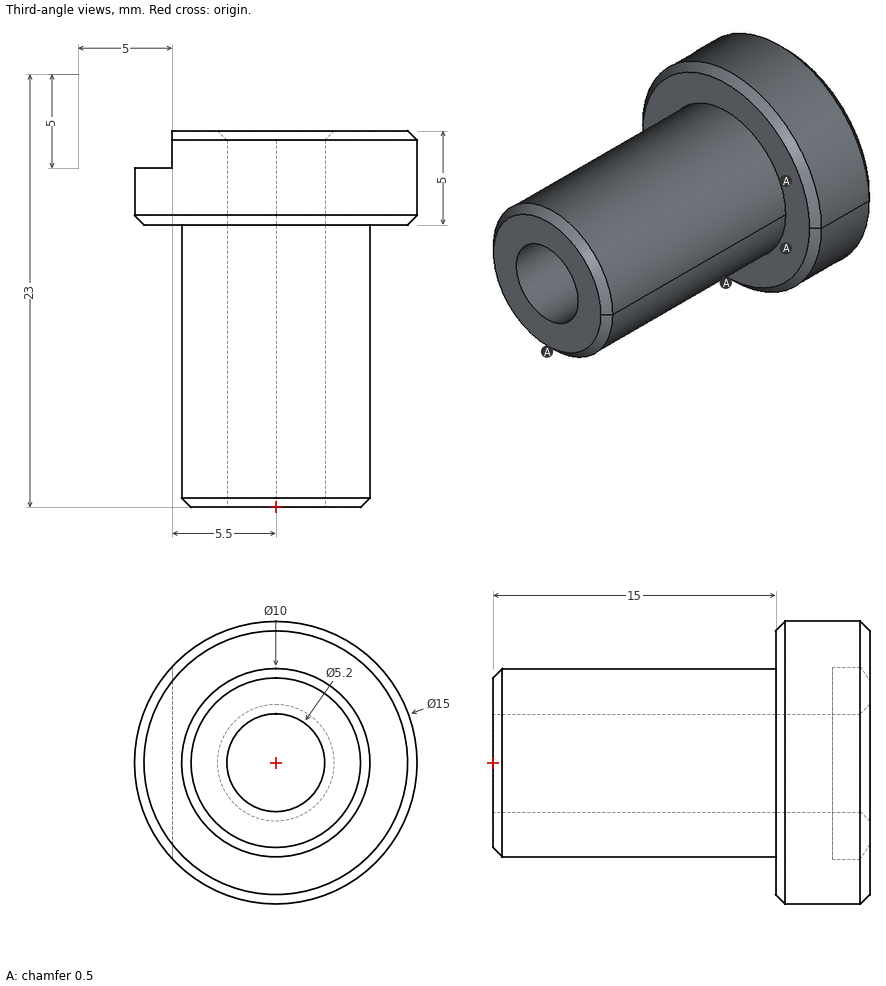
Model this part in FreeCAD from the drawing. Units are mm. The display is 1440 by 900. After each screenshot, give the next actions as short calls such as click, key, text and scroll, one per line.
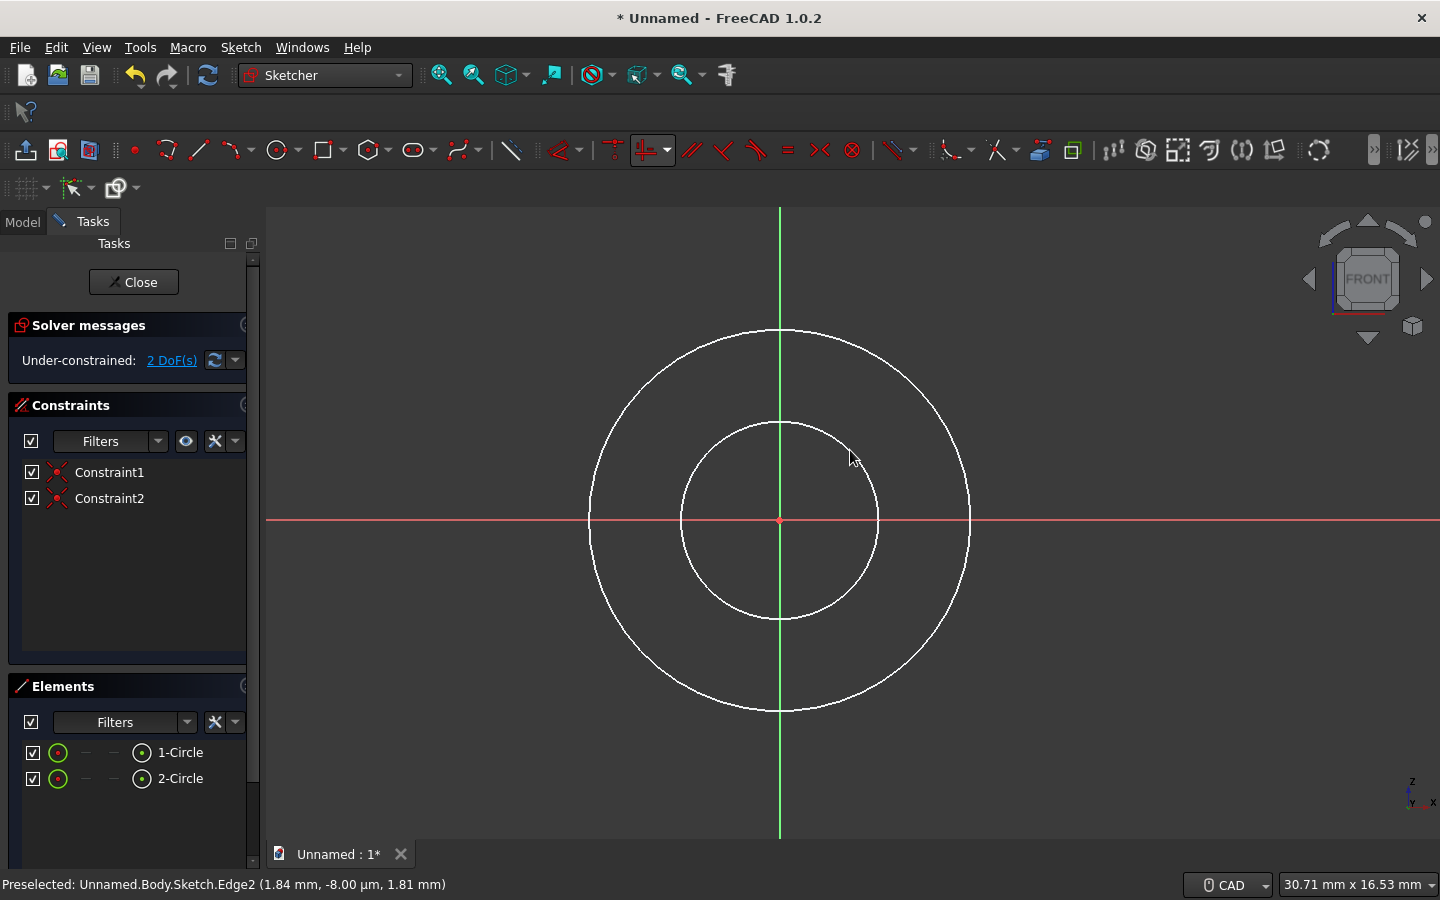
click(914, 385)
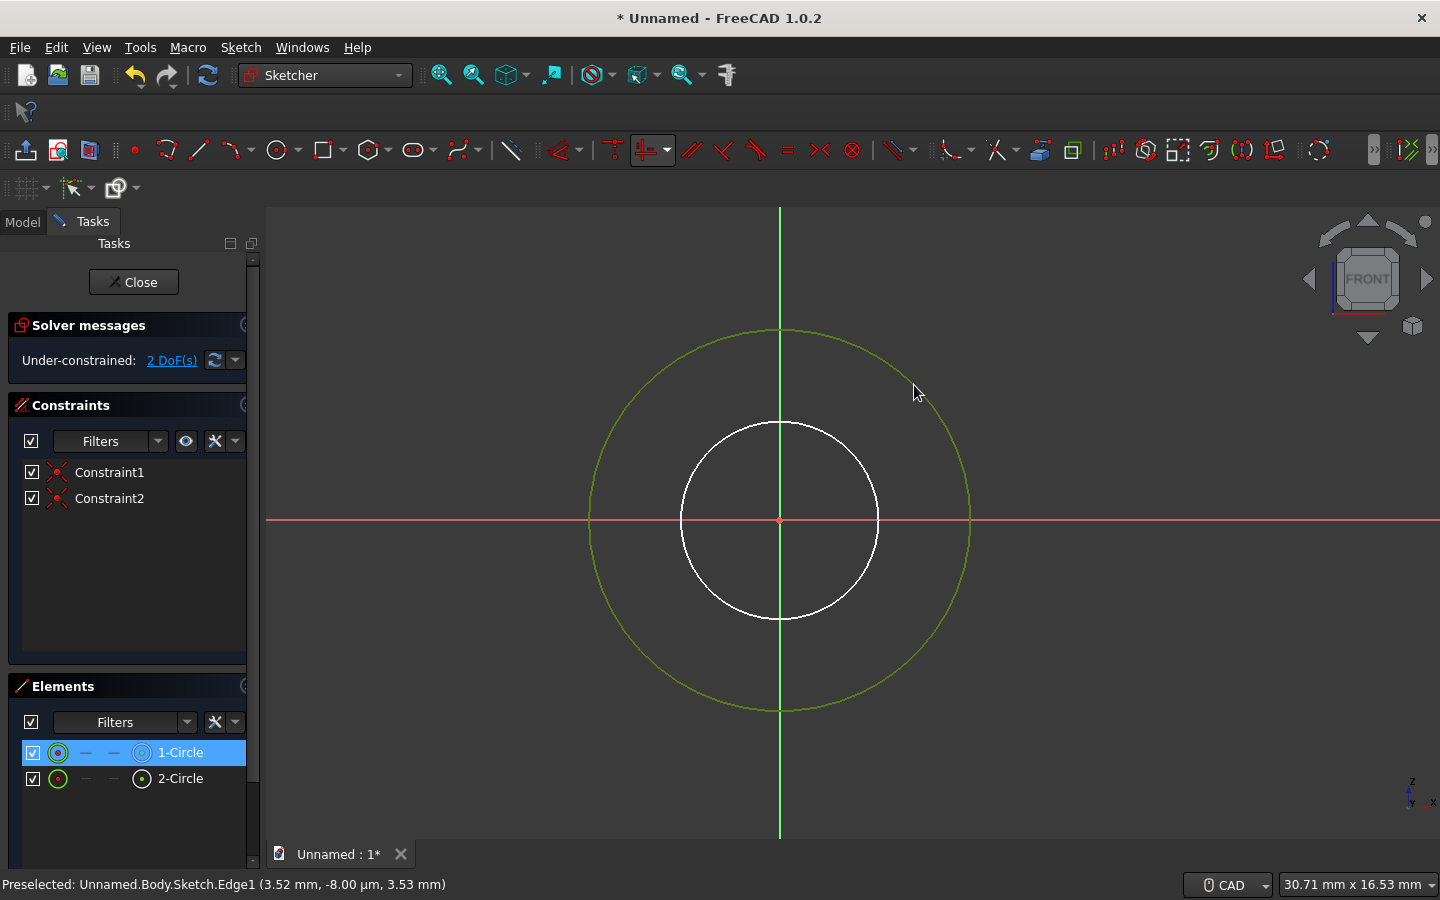
click(582, 150)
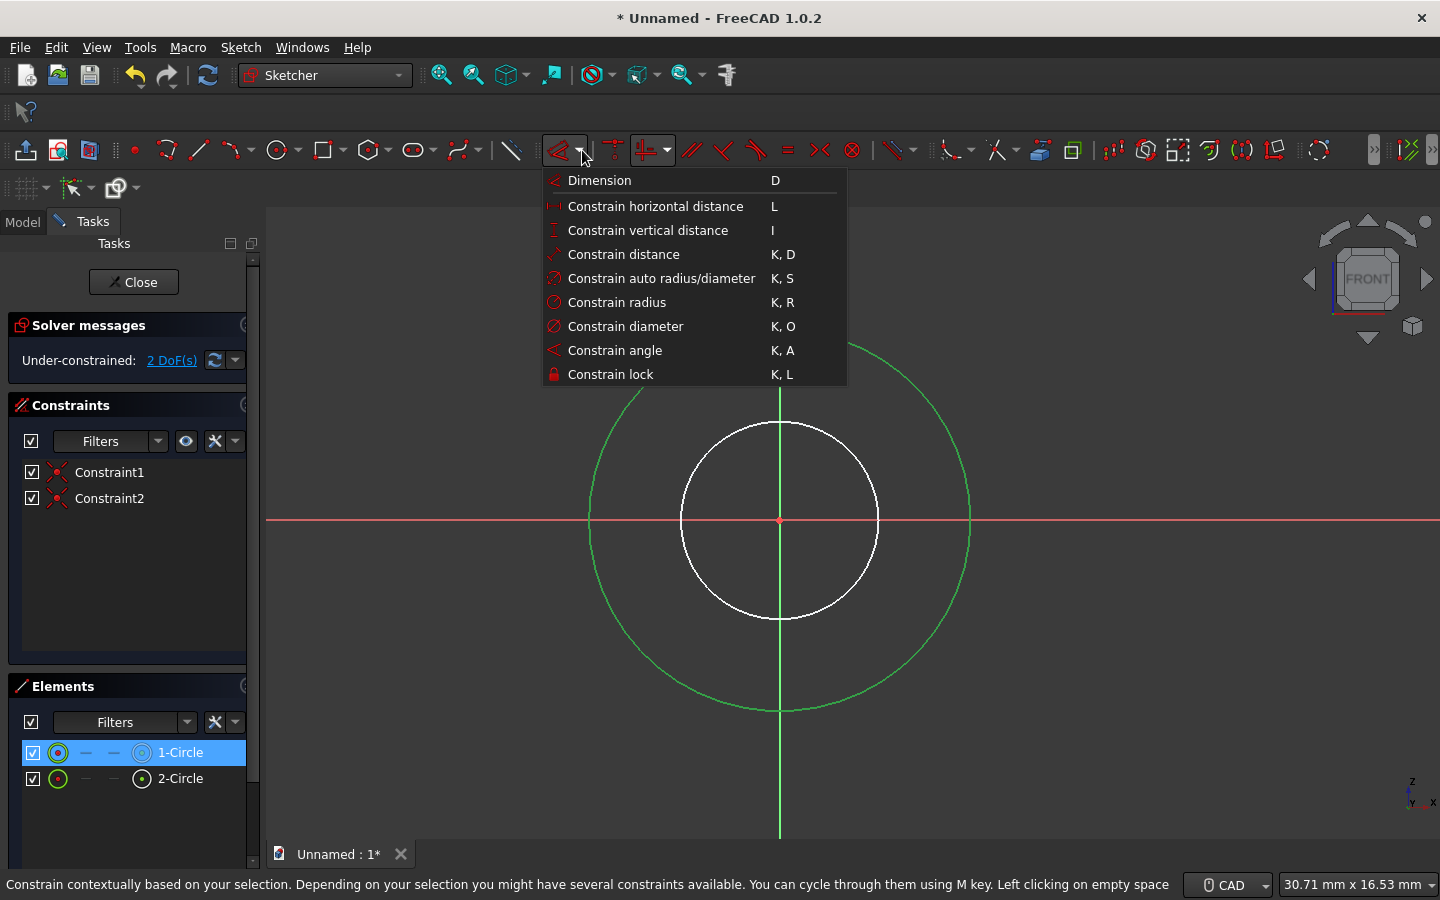
click(695, 326)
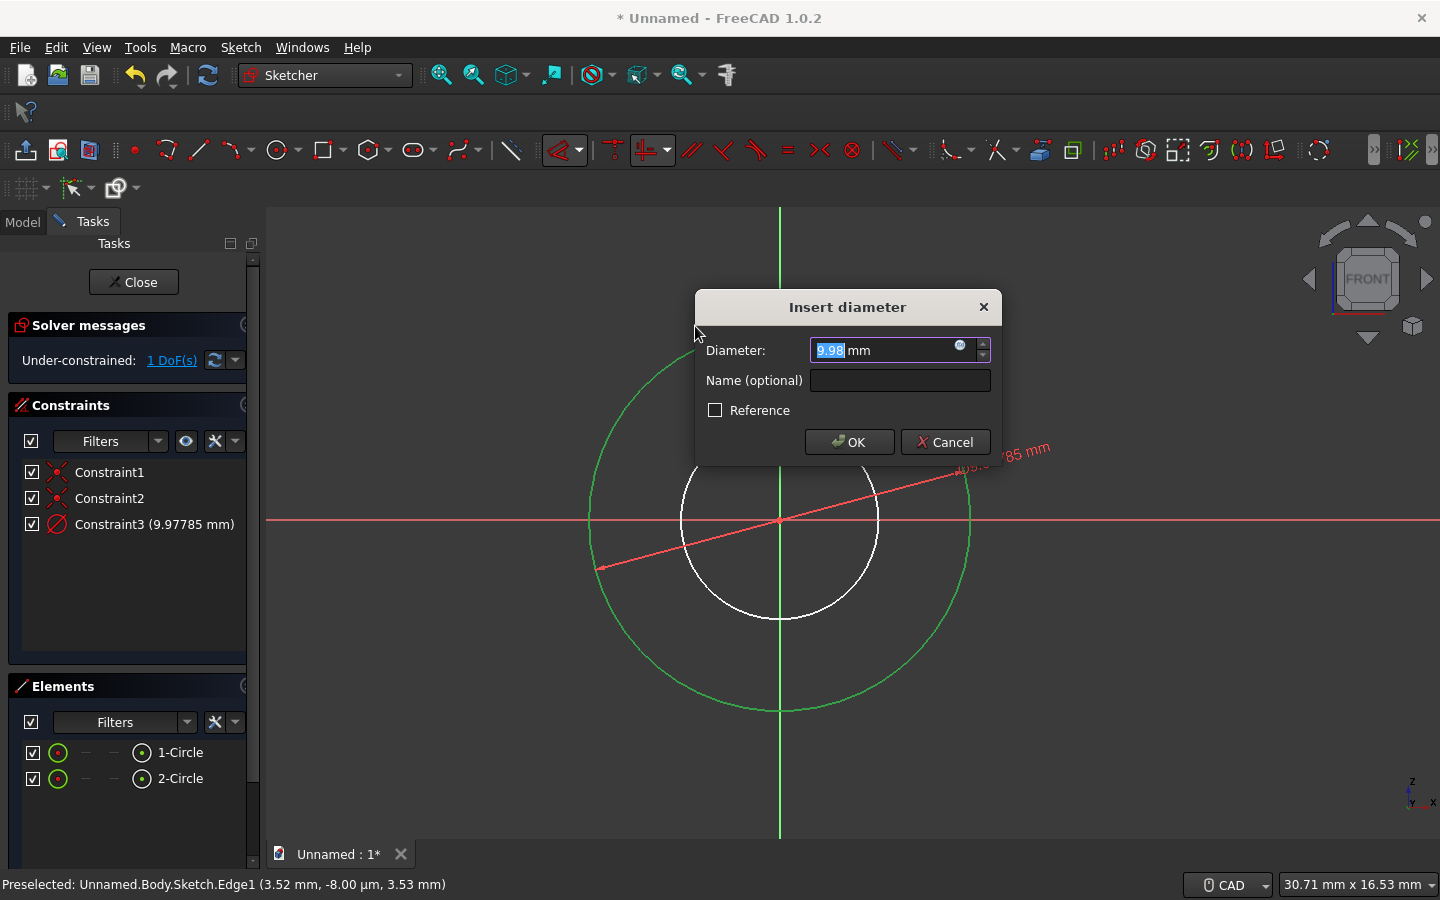
text(10)
key(Return)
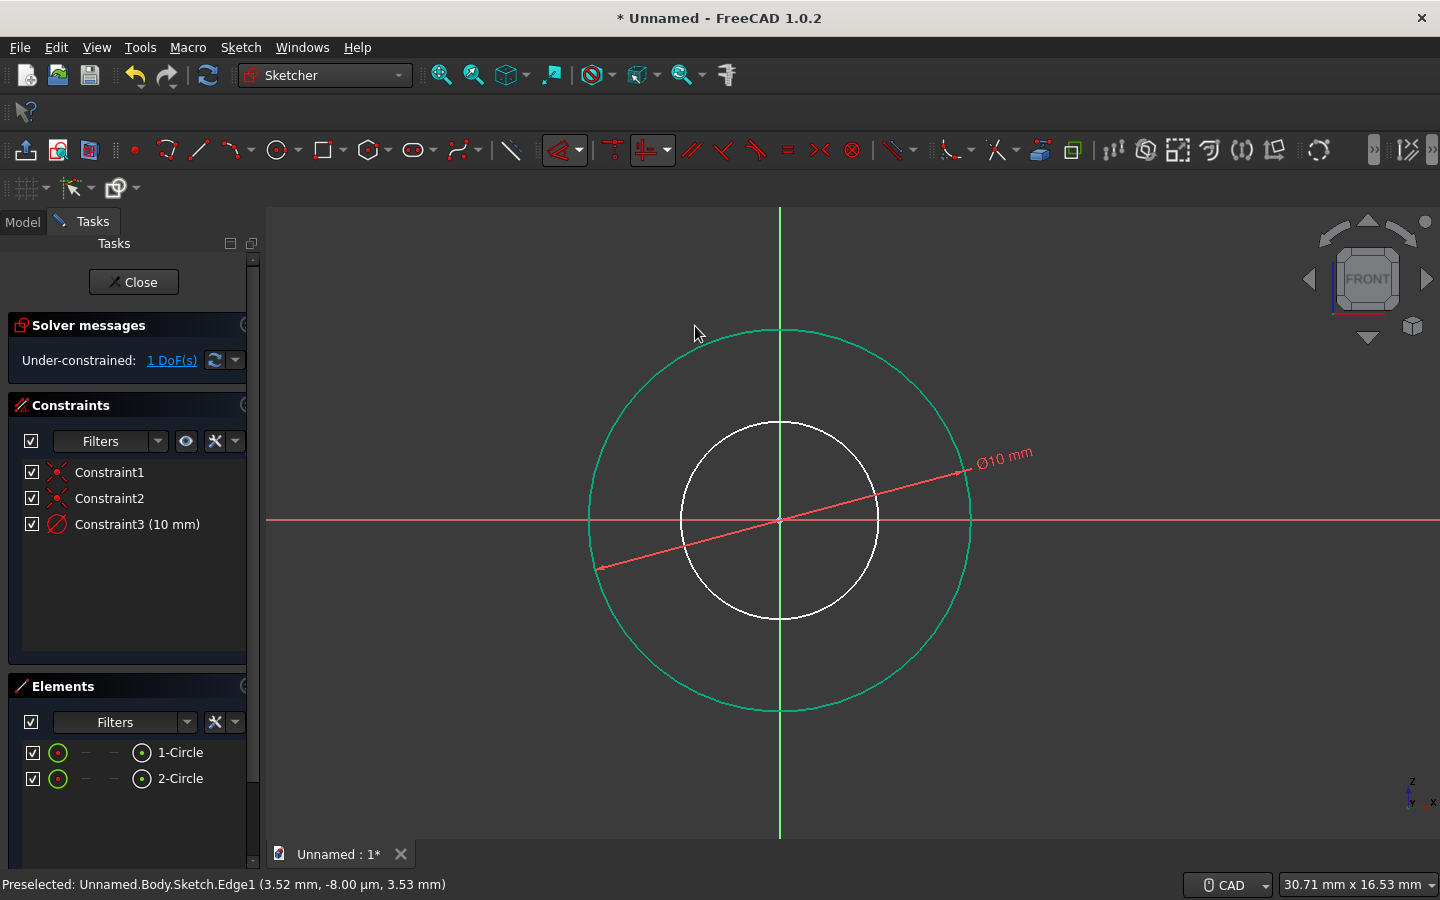
click(849, 450)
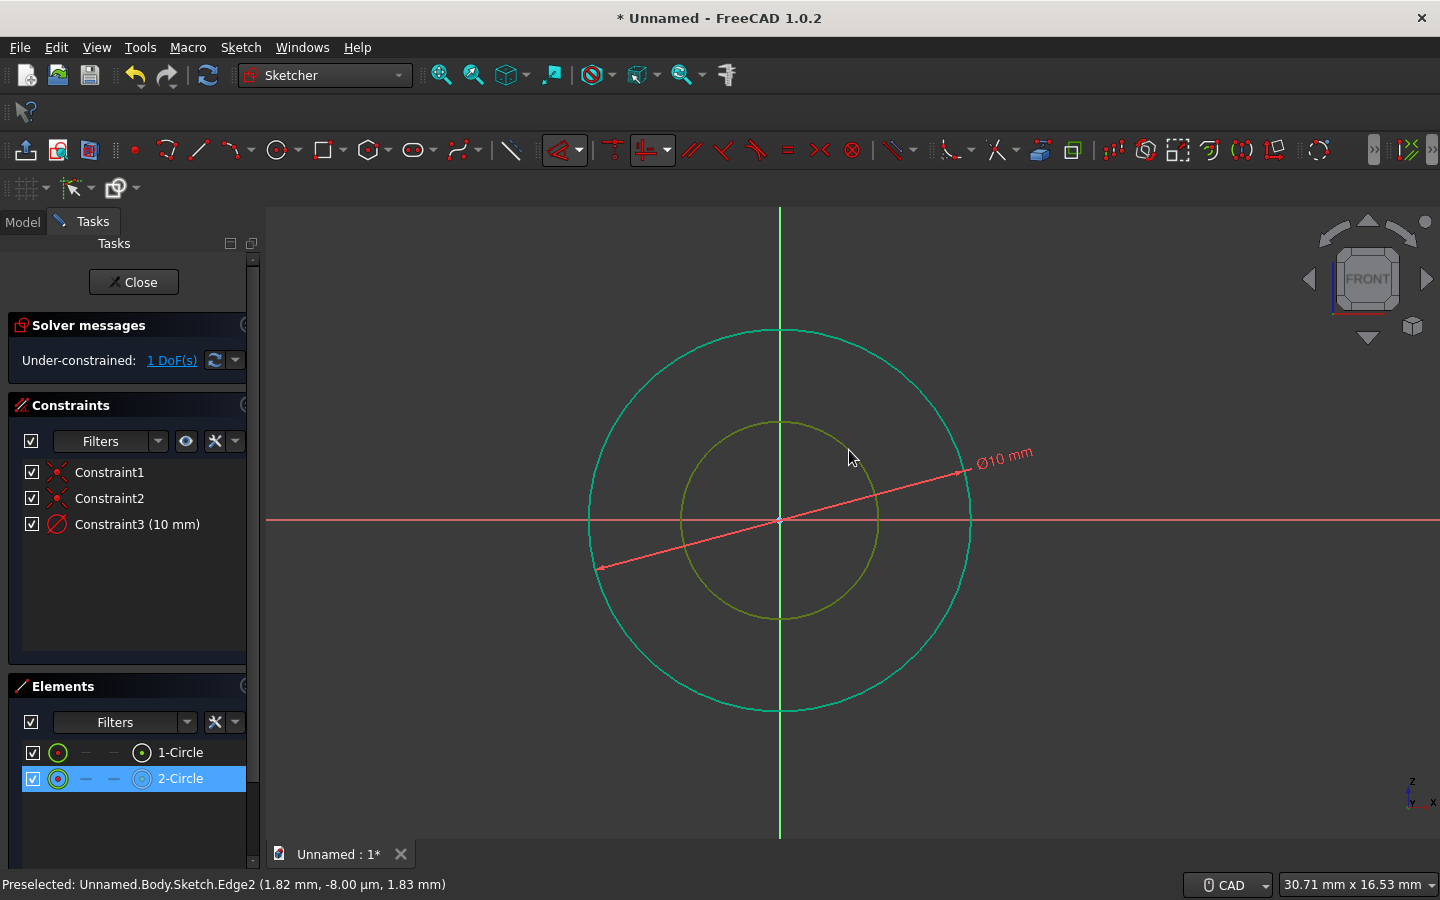
click(582, 150)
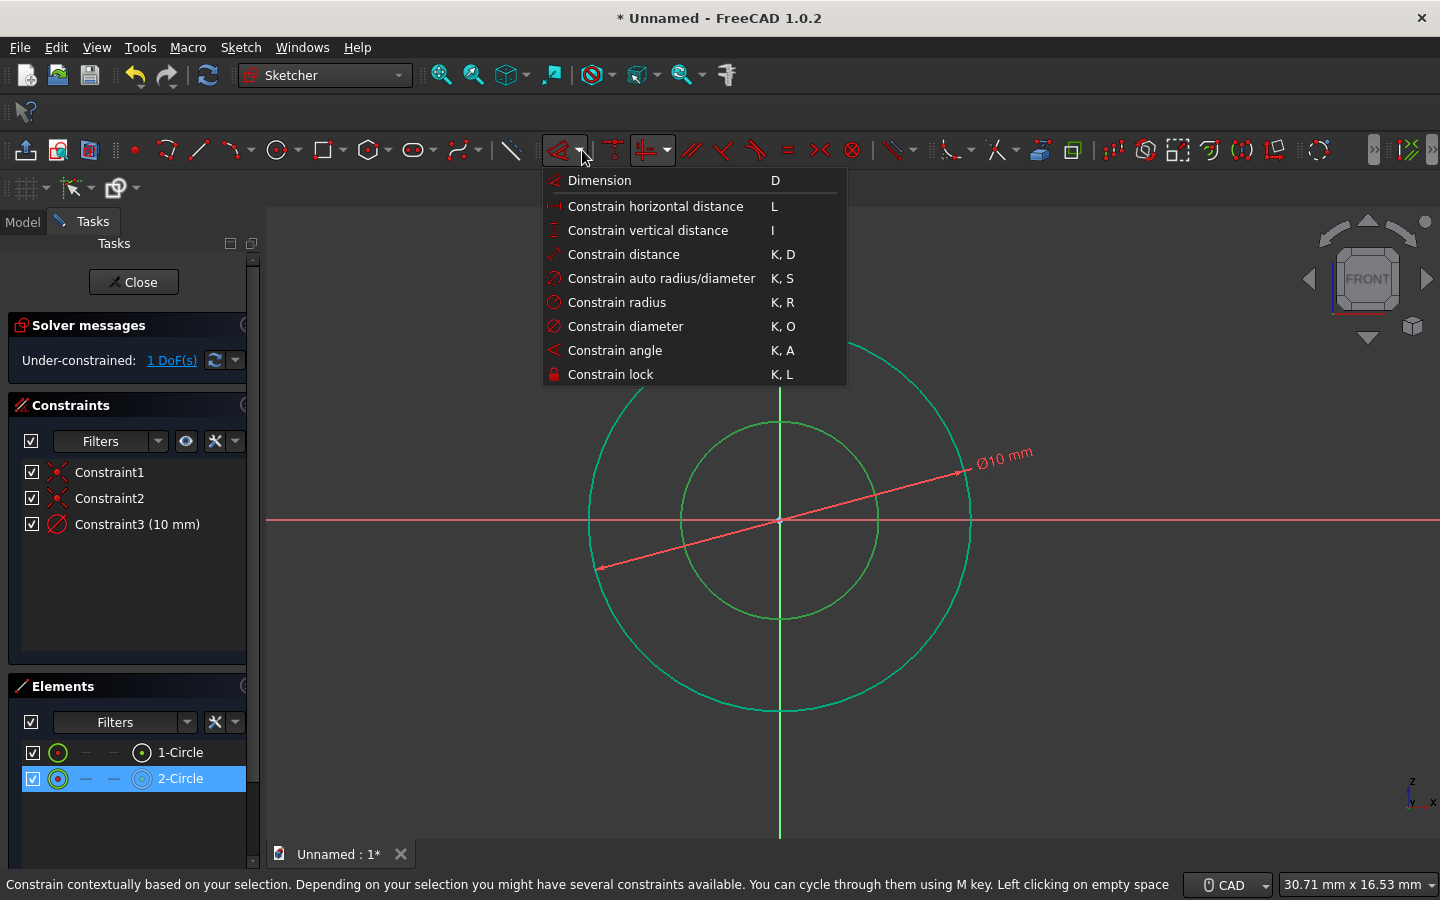
click(695, 326)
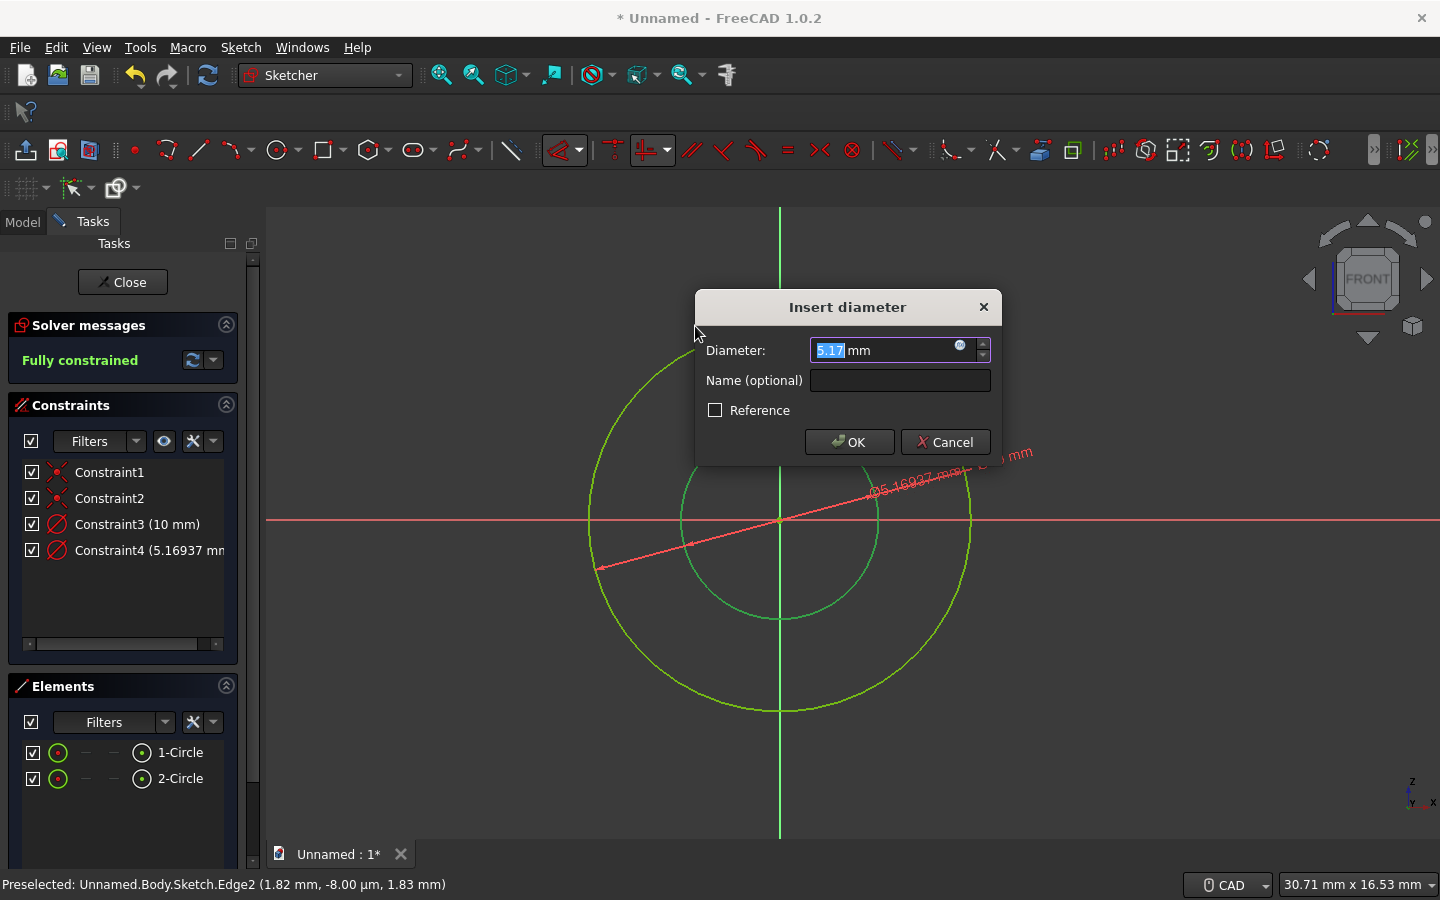
text(5.2)
key(Return)